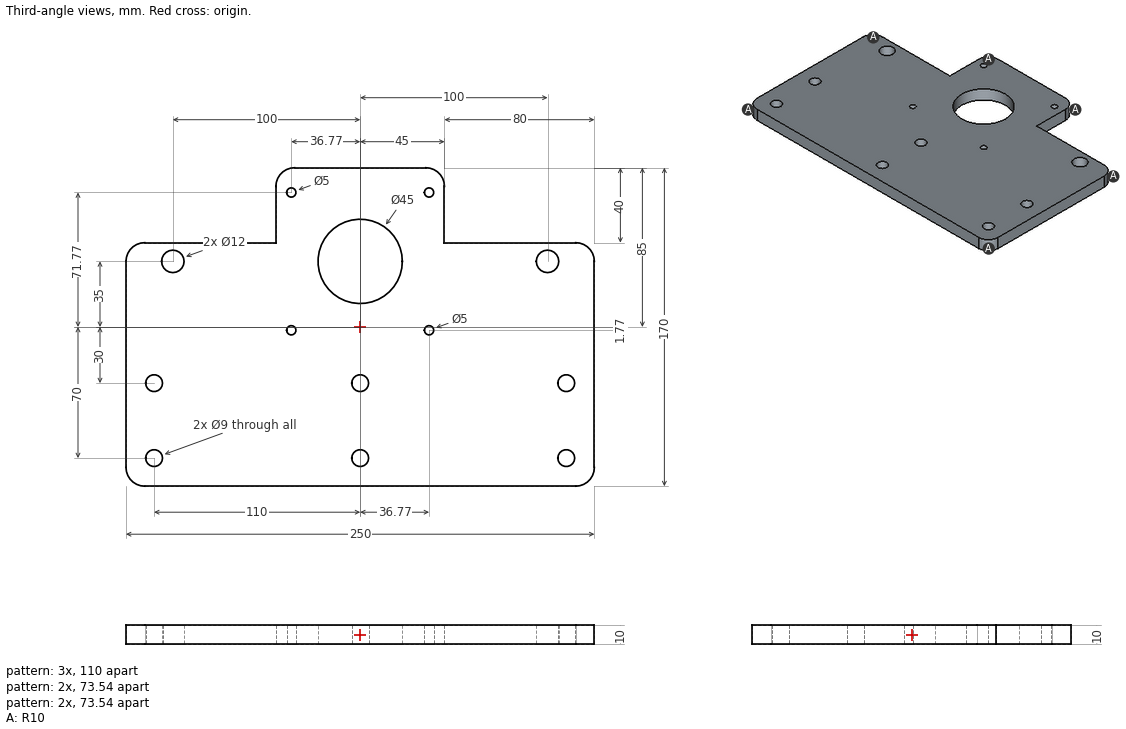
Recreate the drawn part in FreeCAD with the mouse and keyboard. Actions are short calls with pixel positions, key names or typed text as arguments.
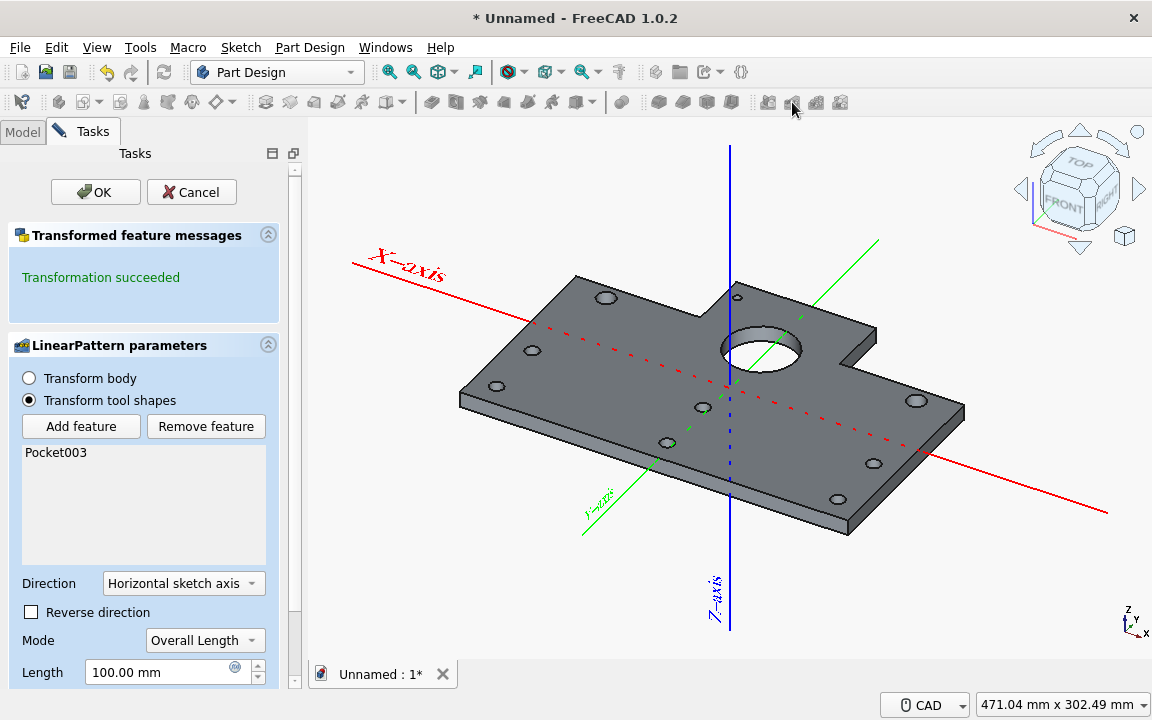
click(184, 584)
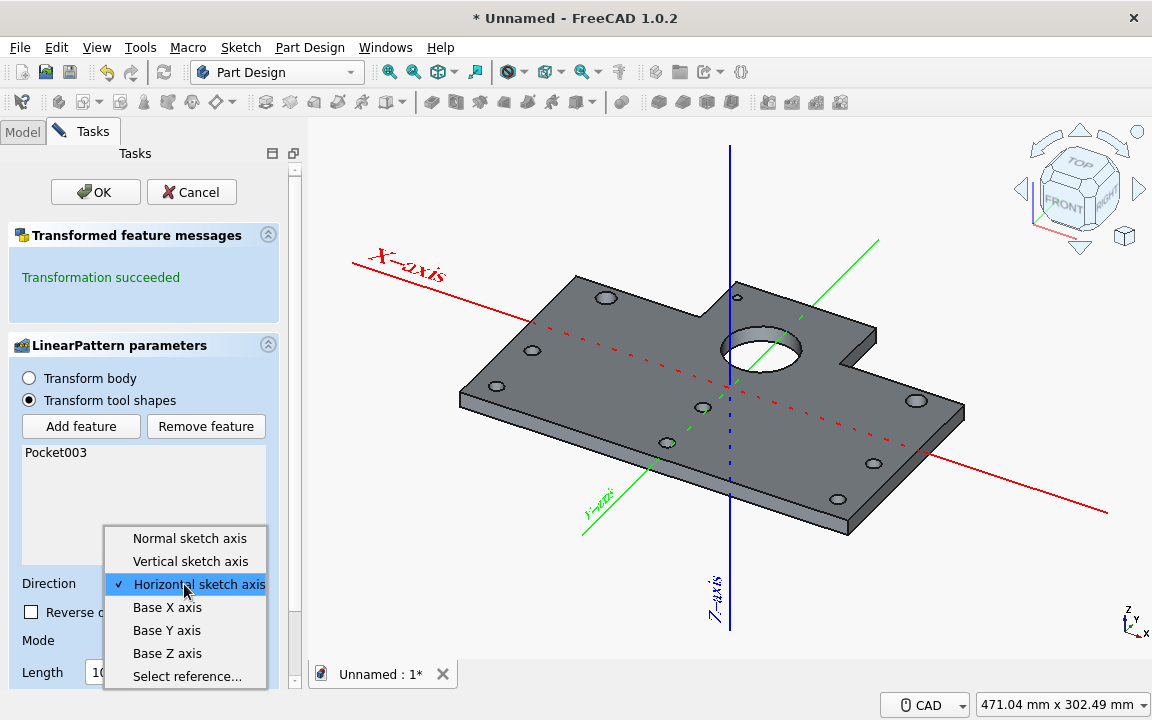
click(184, 630)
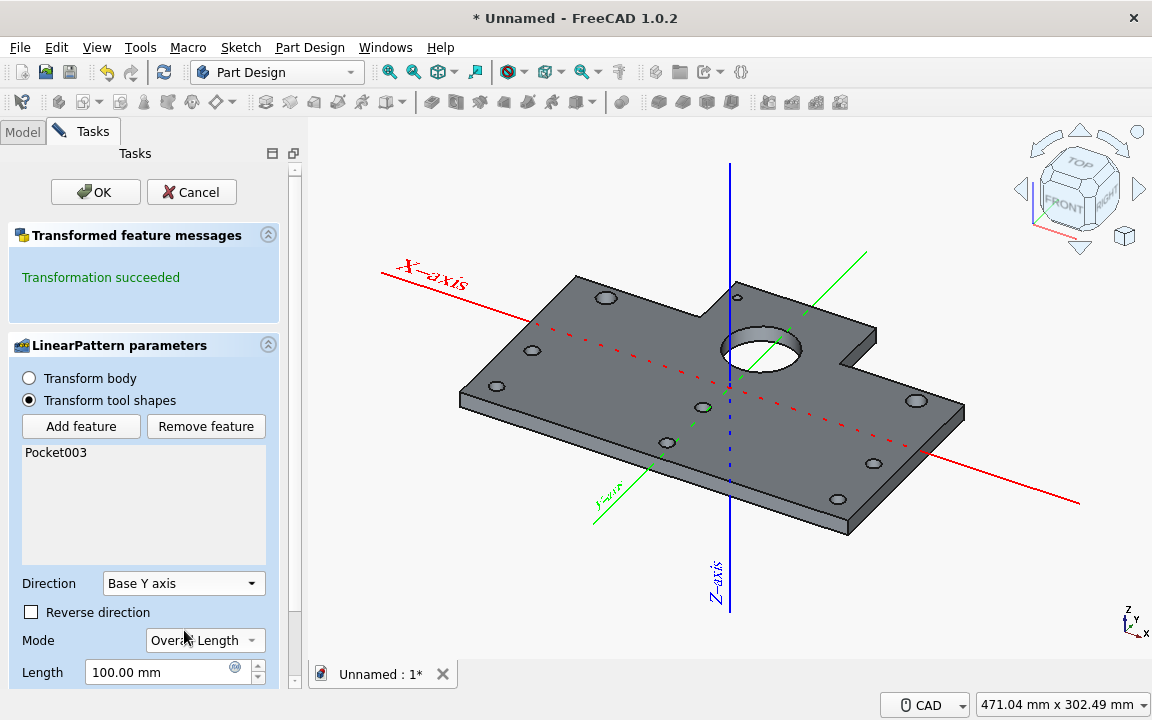
click(206, 640)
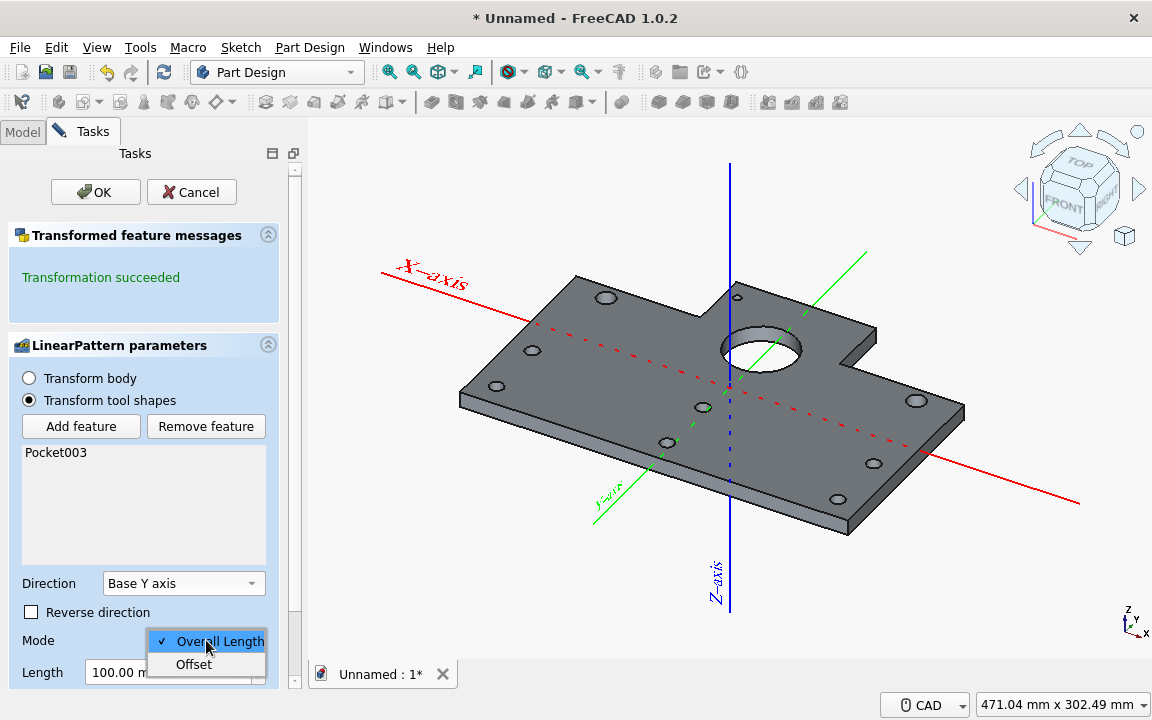
click(206, 664)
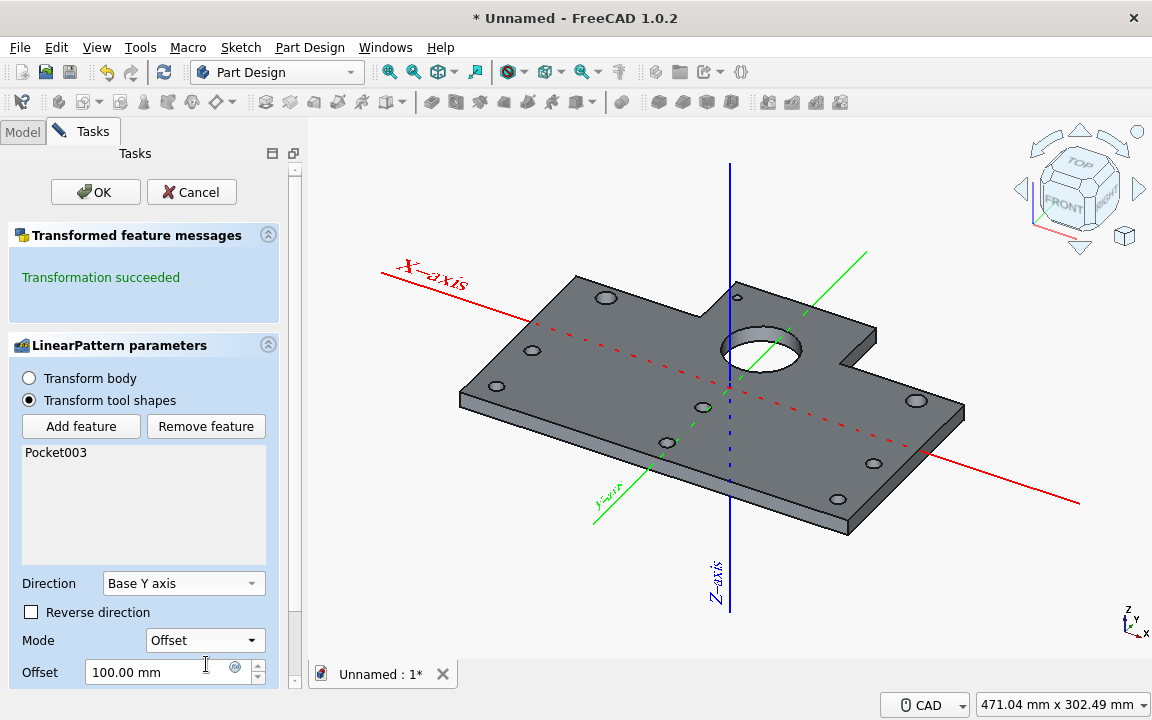
triple_click(168, 672)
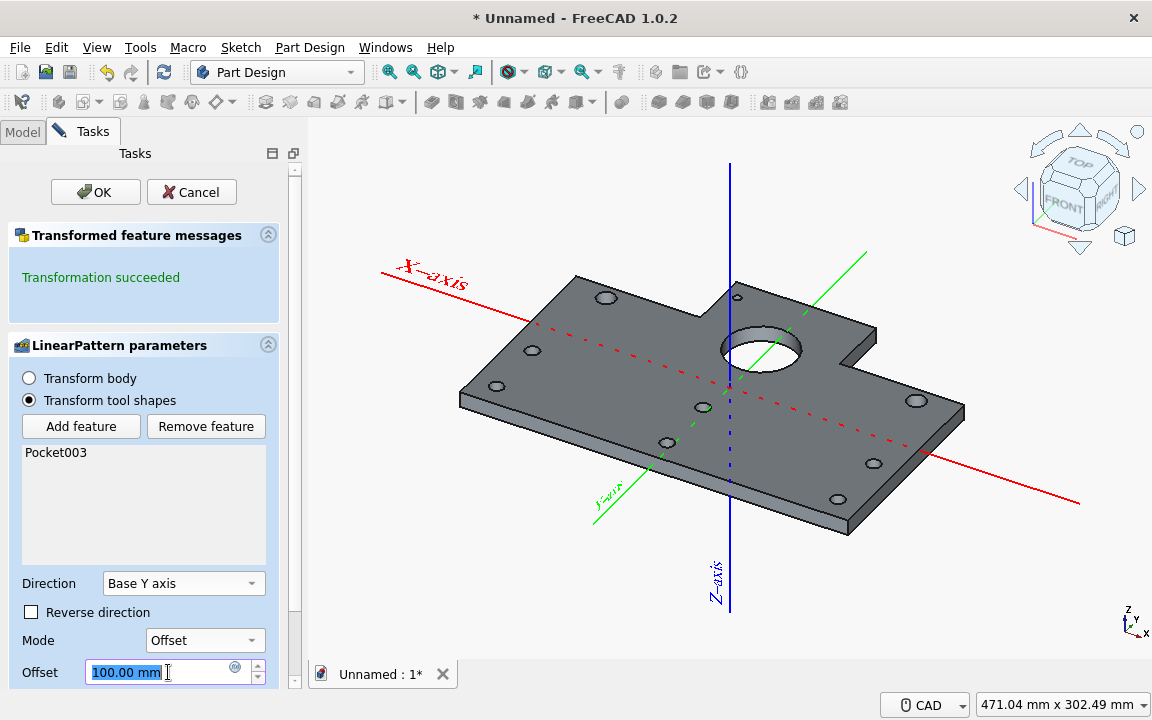
text(73.54)
key(Tab)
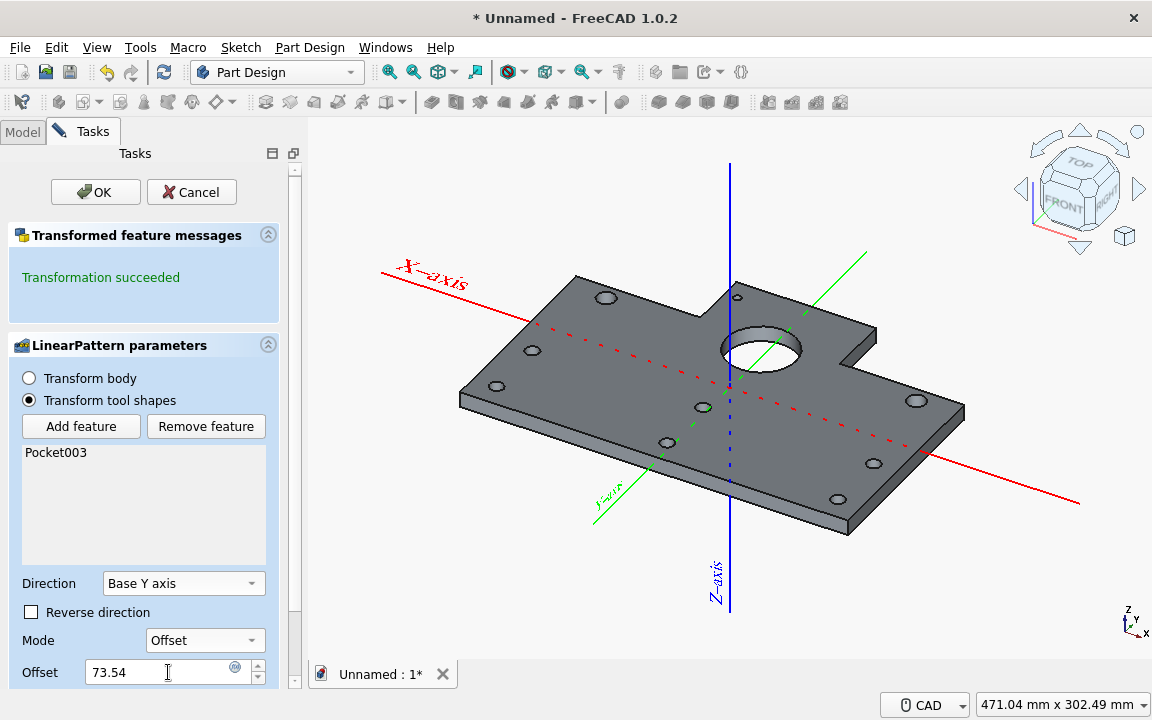
scroll(295, 426, down, 2)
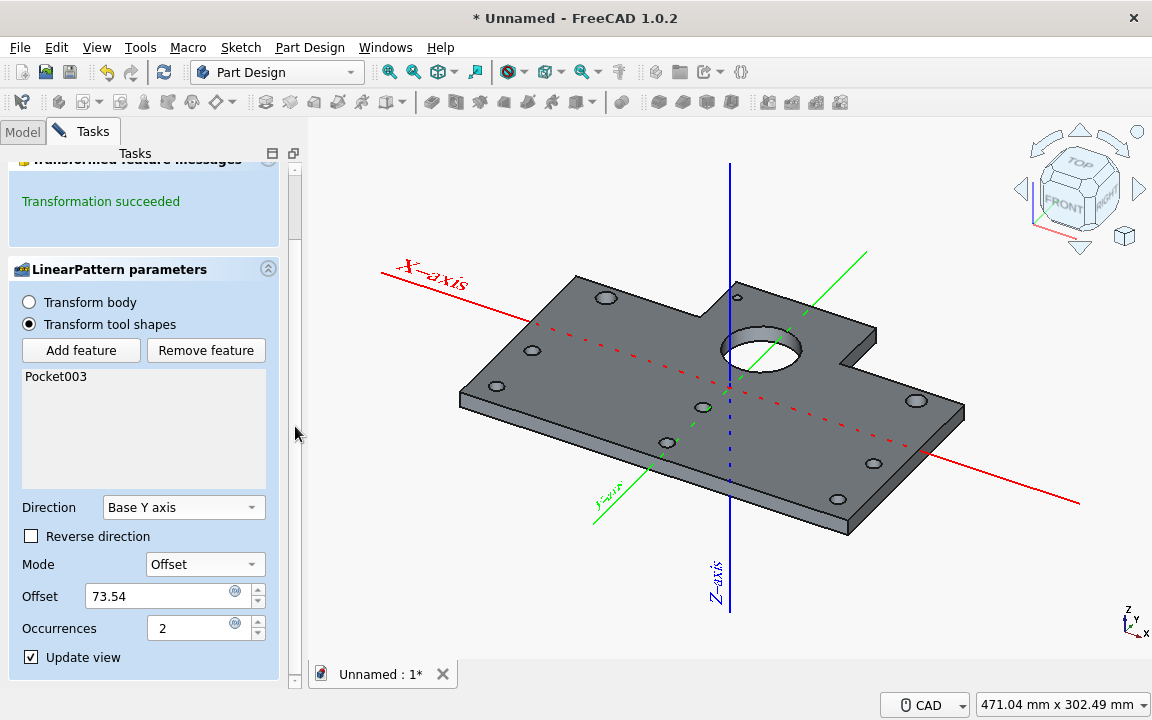
triple_click(198, 628)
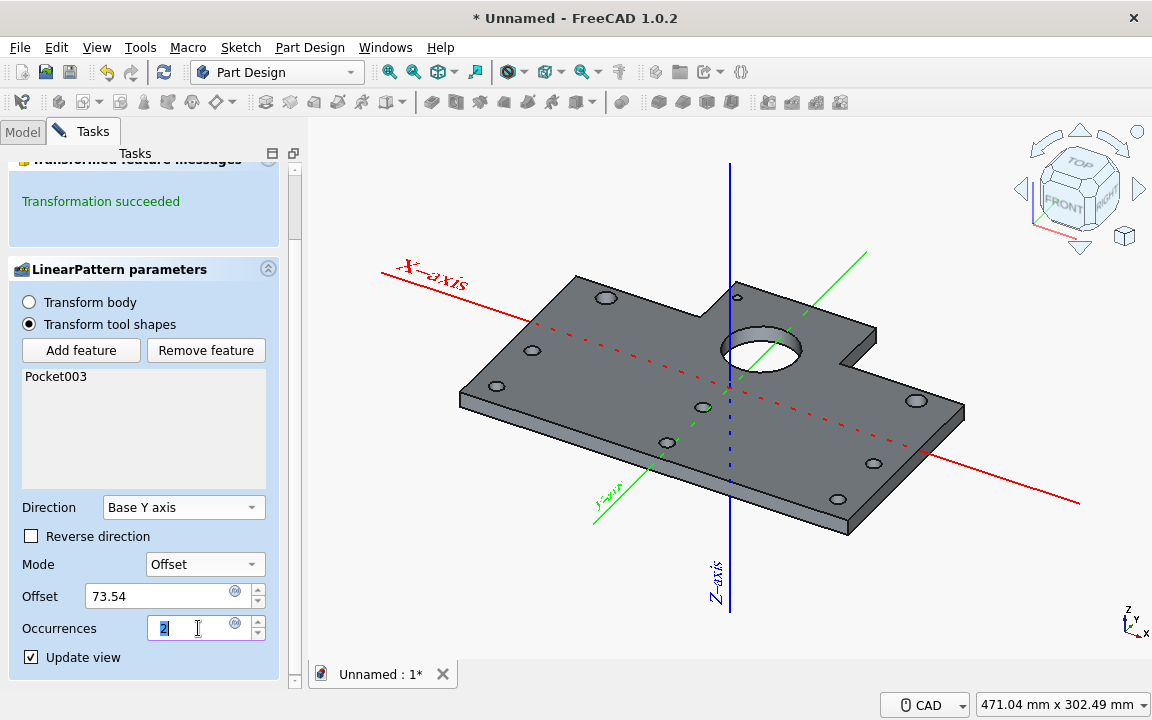
text(2)
key(Tab)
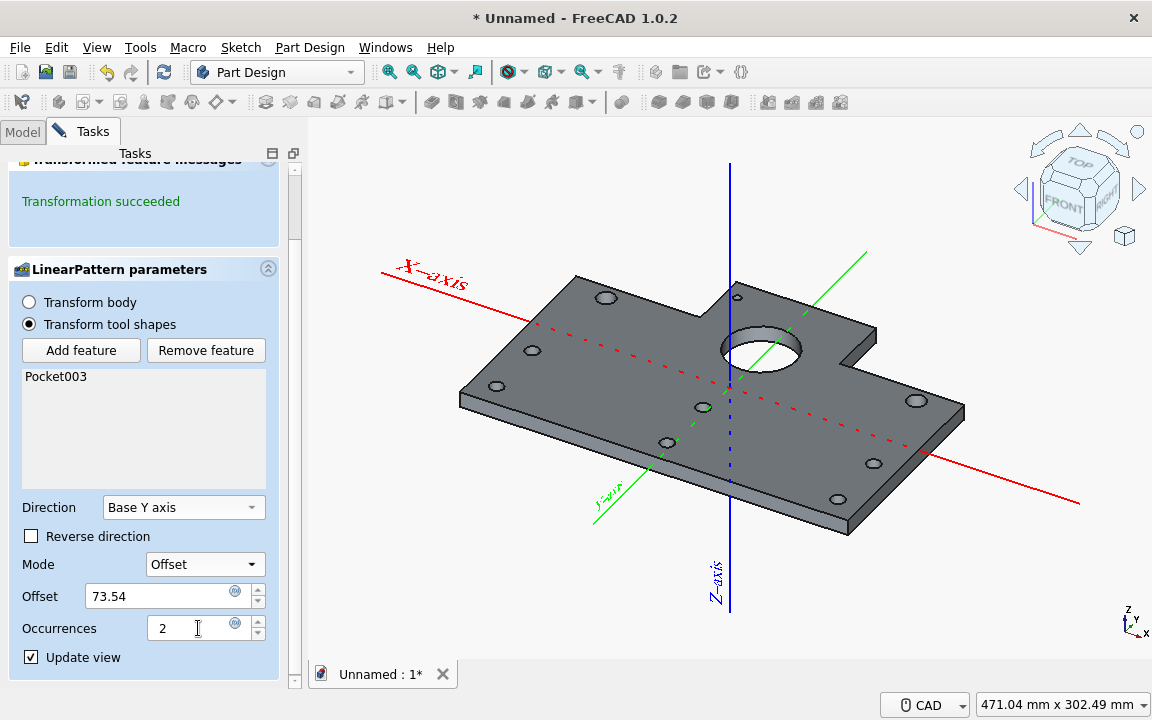
click(30, 536)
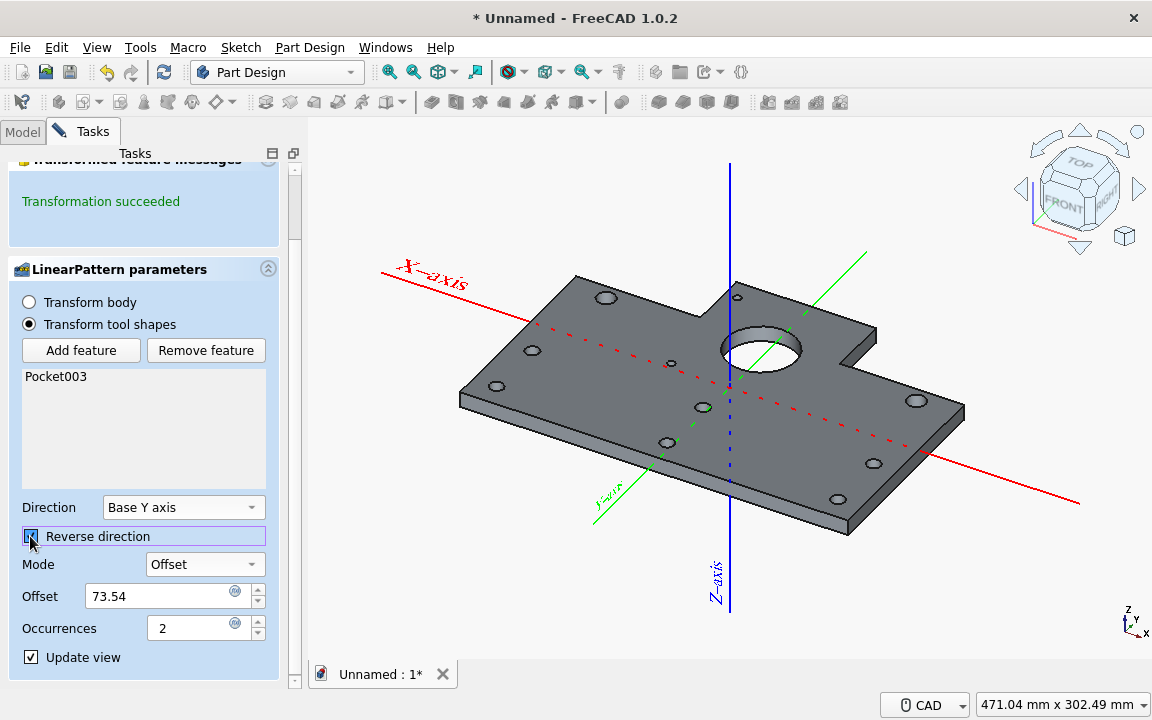
scroll(295, 426, up, 3)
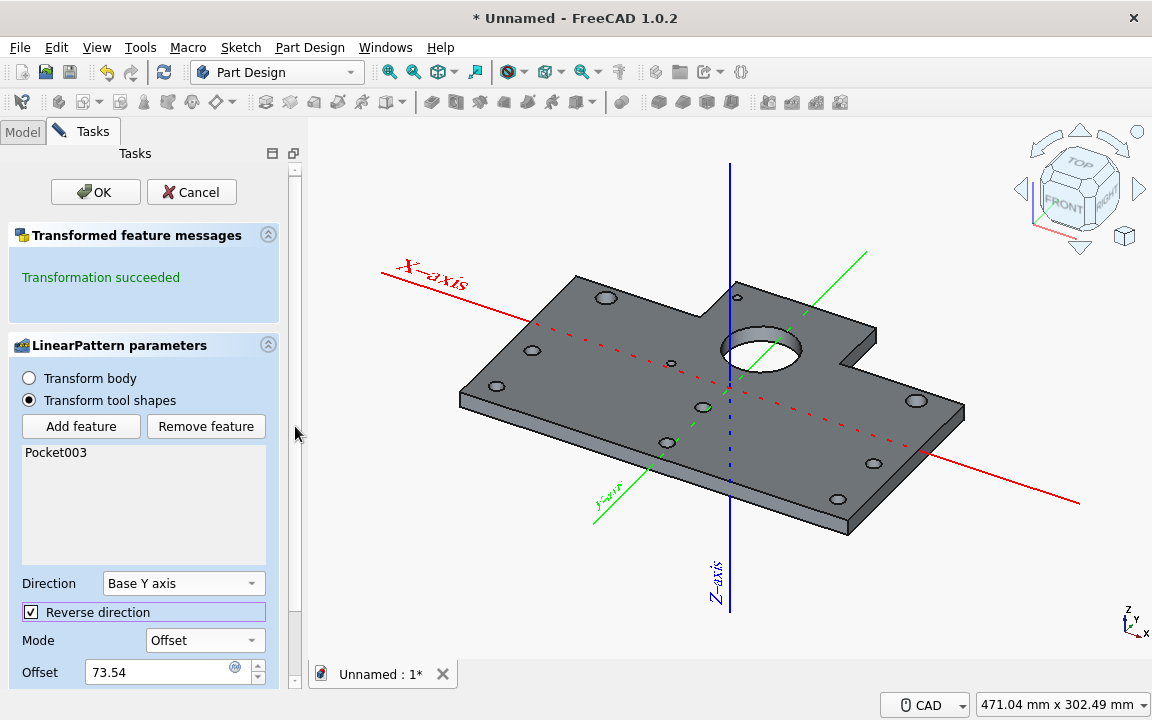
click(96, 192)